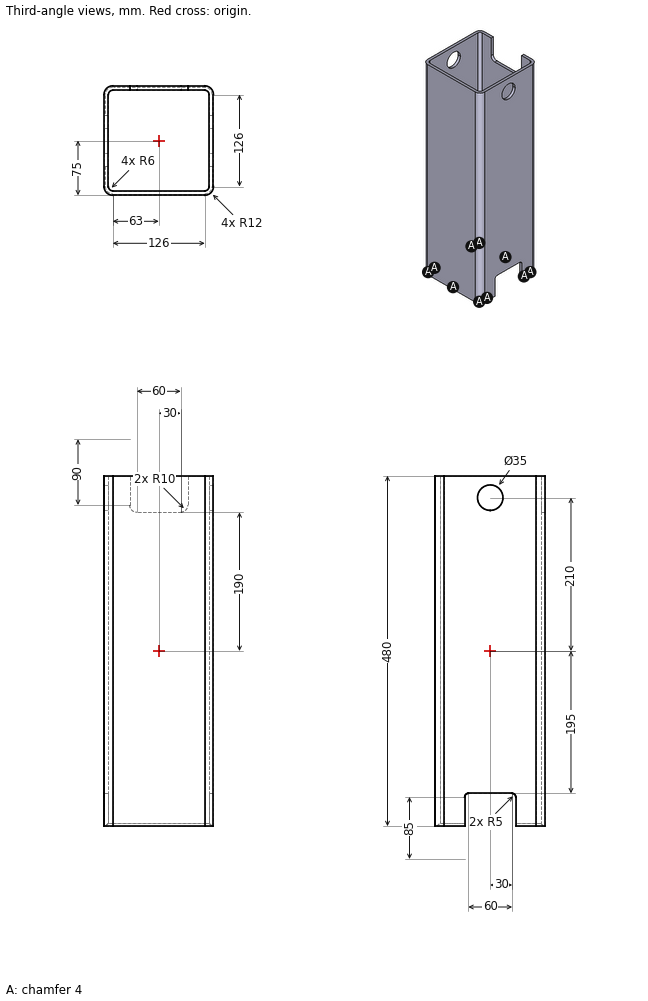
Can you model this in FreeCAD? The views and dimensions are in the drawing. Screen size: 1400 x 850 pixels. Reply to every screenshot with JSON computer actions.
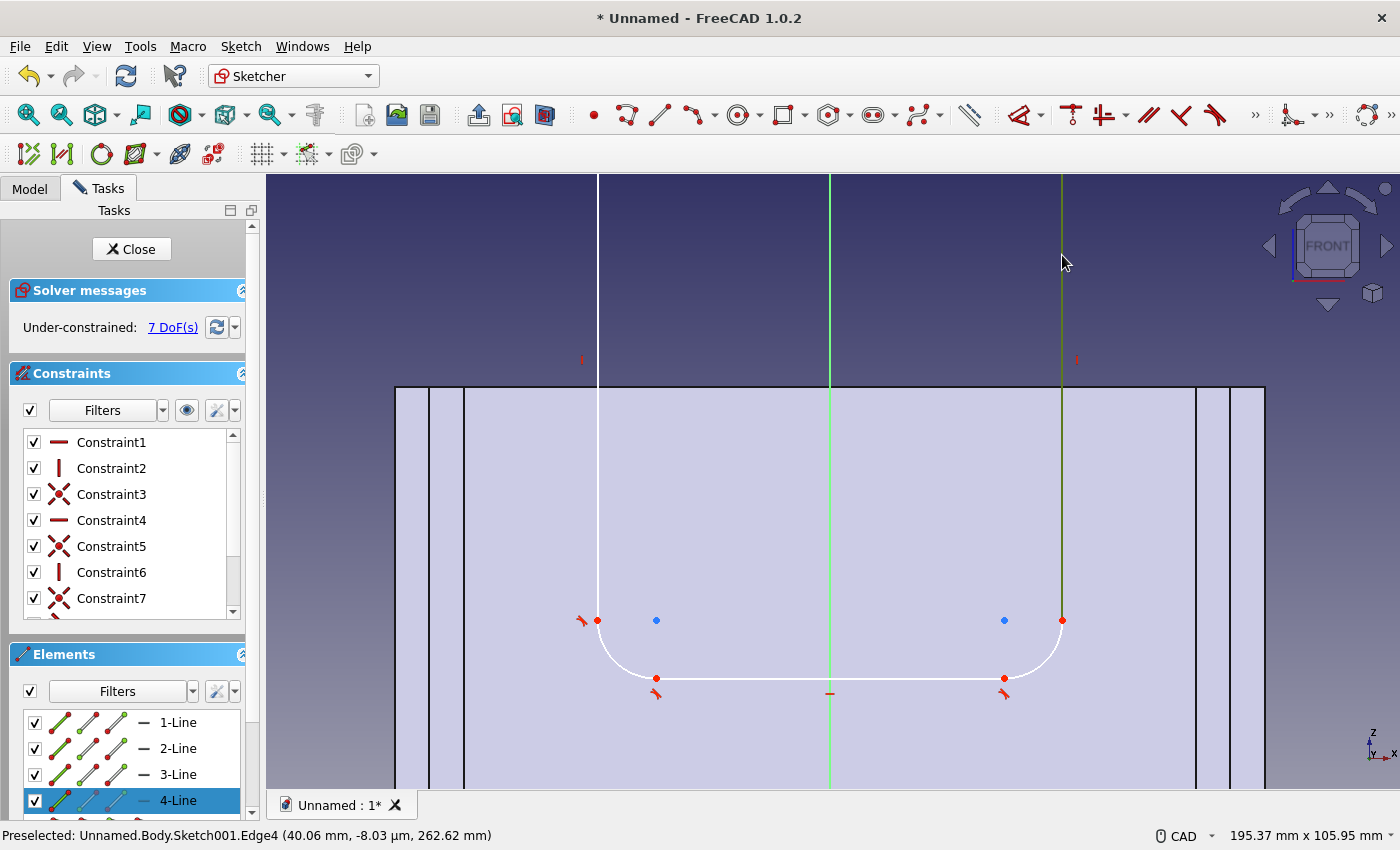
{"action": "left_click", "coordinate": [1031, 672]}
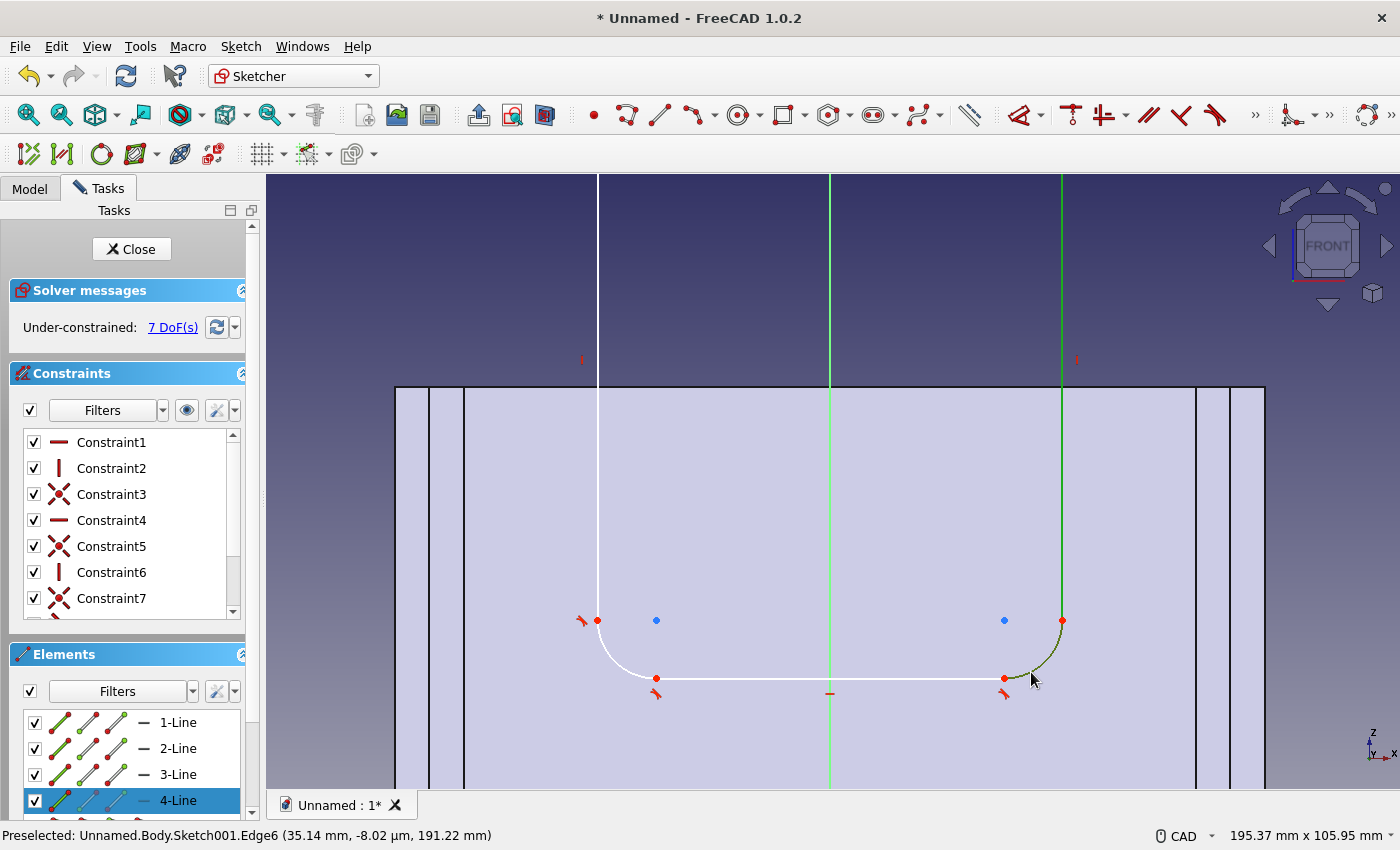
{"action": "key", "text": "t"}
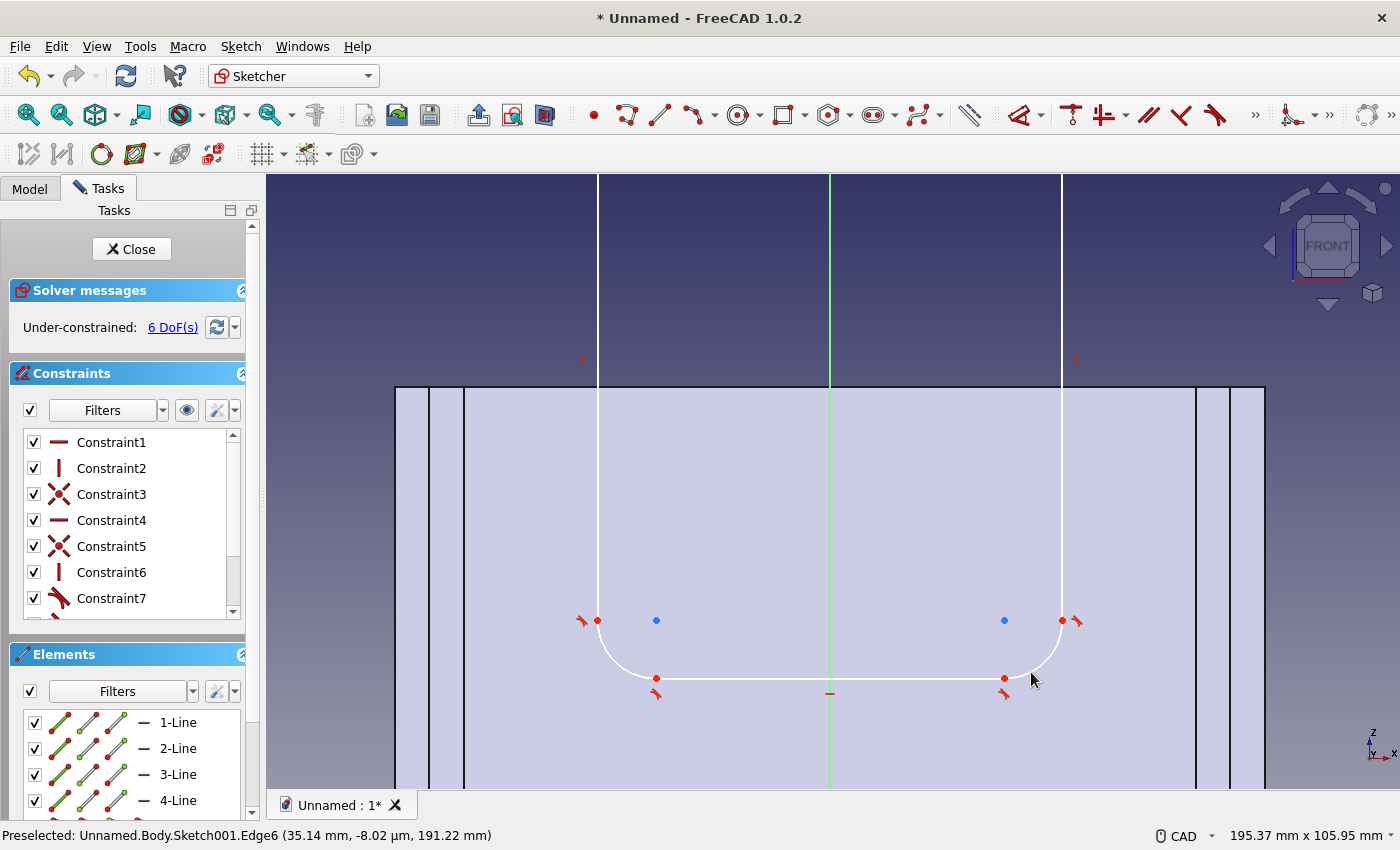
{"action": "left_click", "coordinate": [604, 647]}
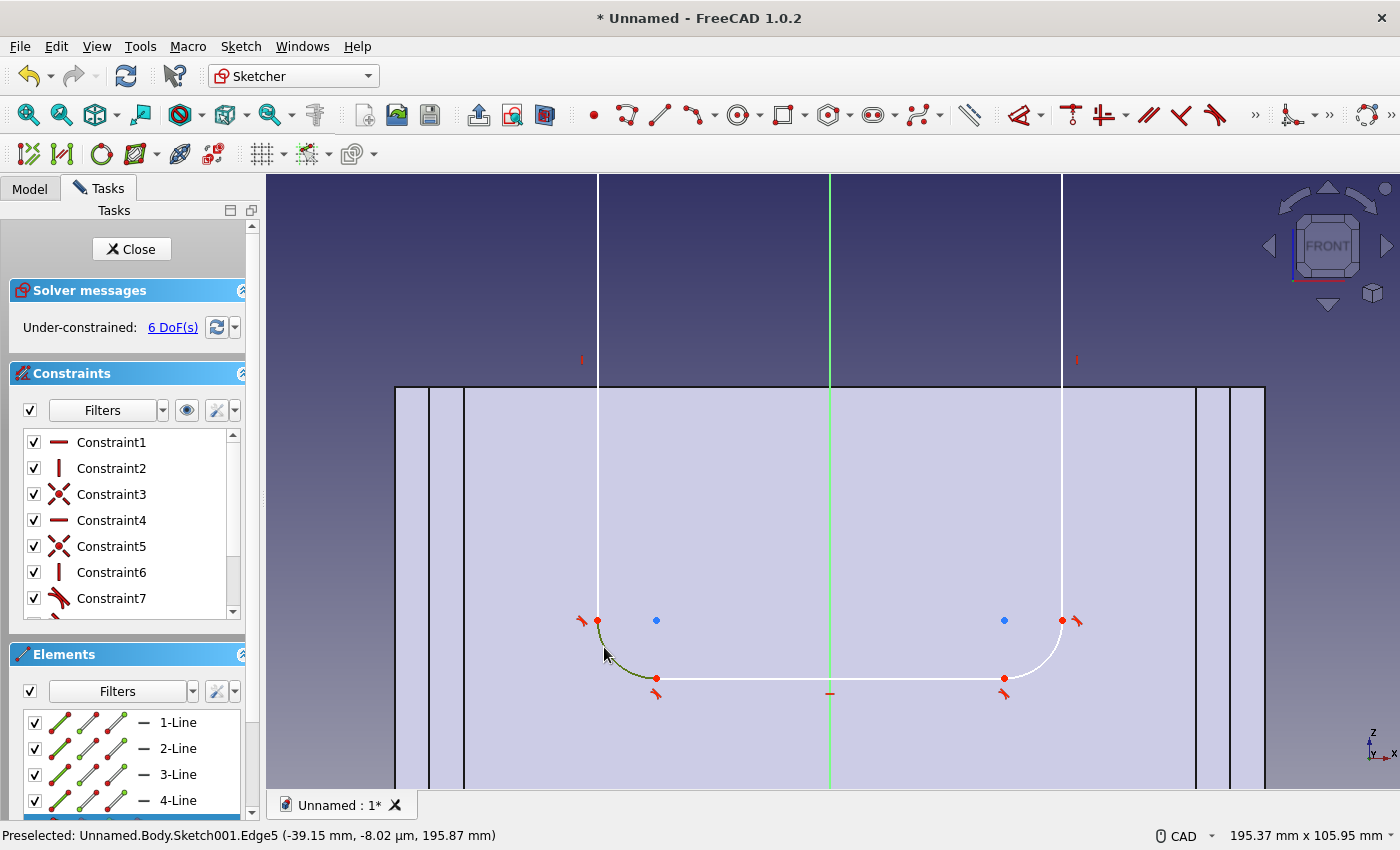
{"action": "left_click", "coordinate": [1031, 672]}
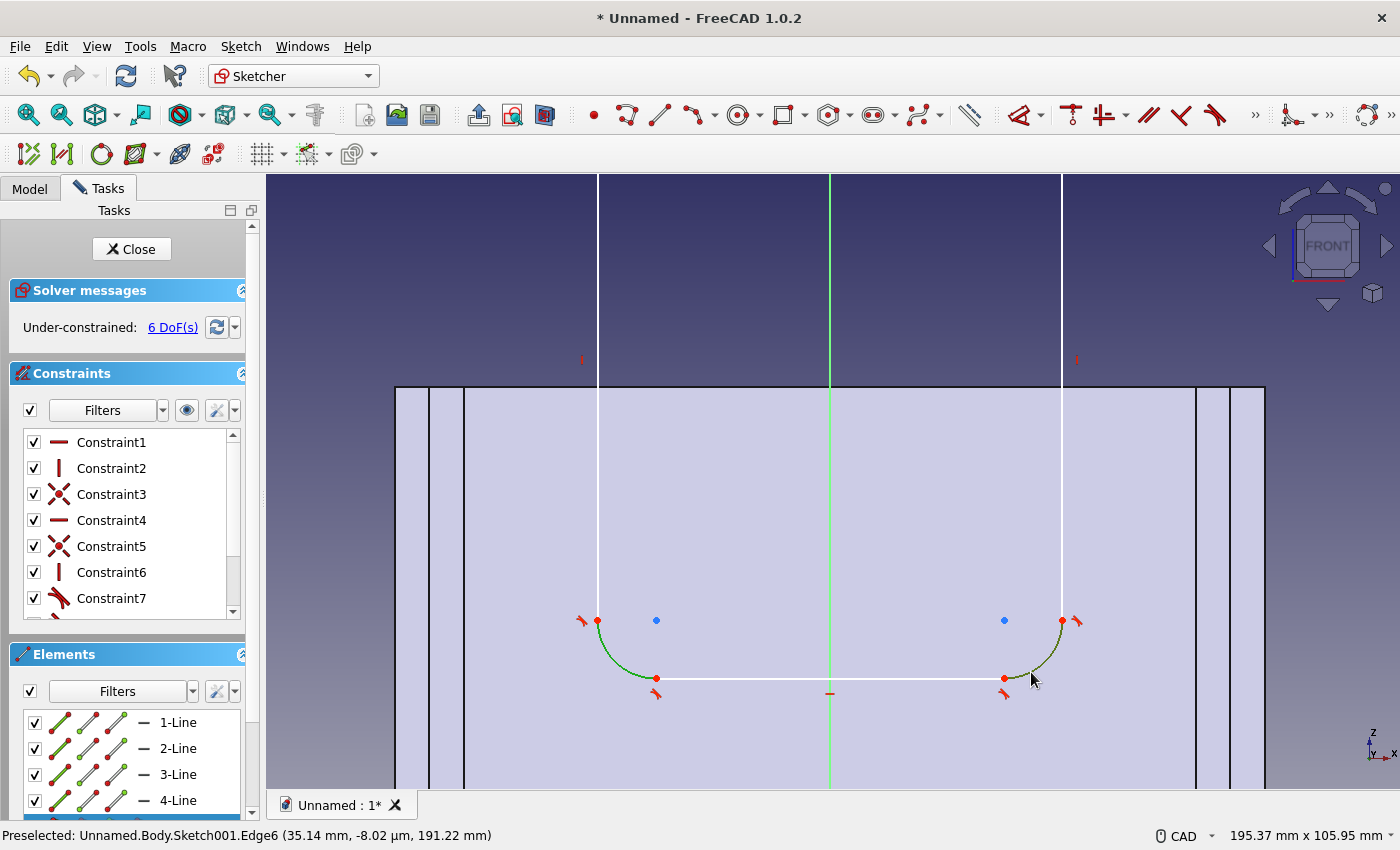
{"action": "key", "text": "e"}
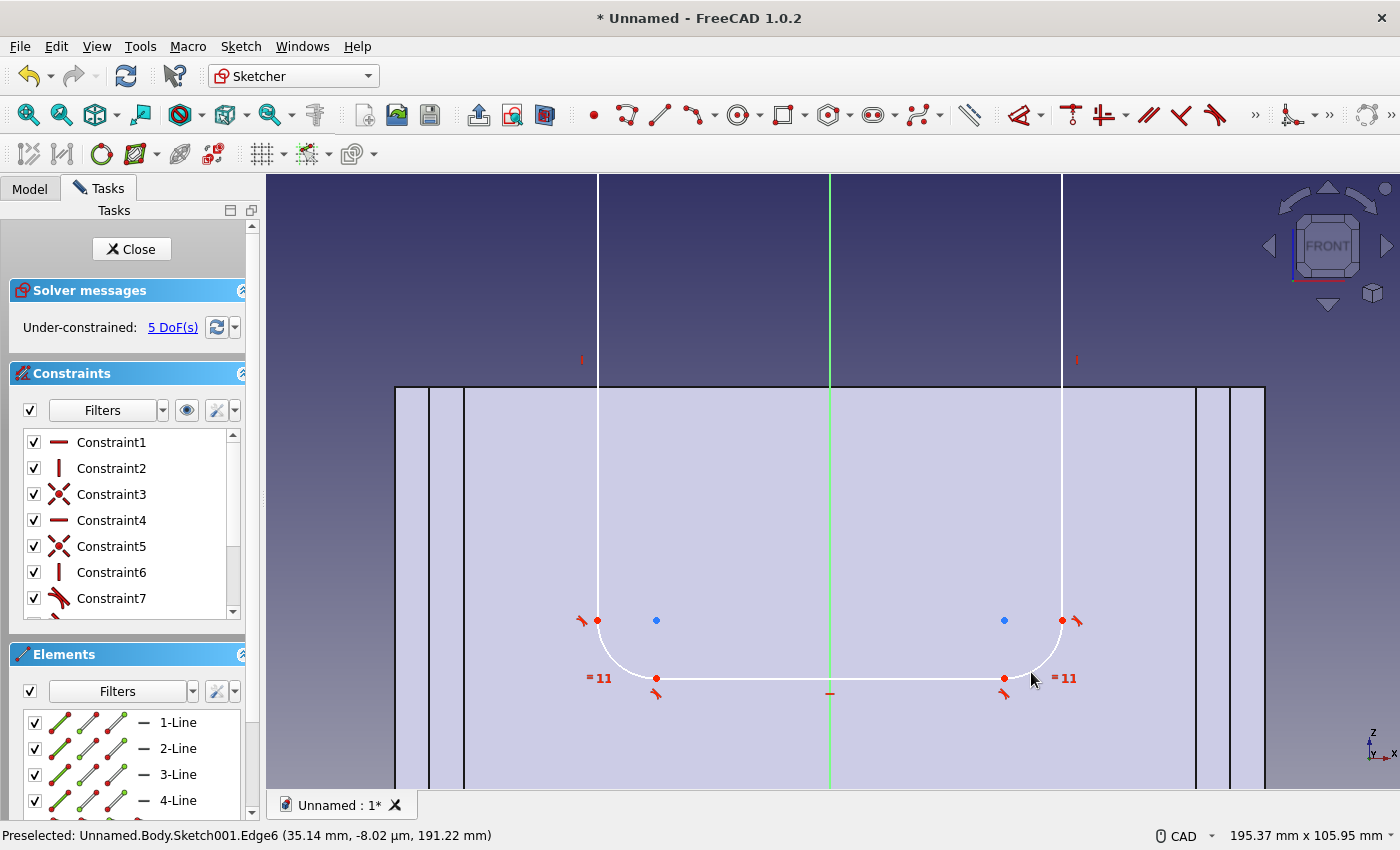
{"action": "left_click", "coordinate": [604, 647]}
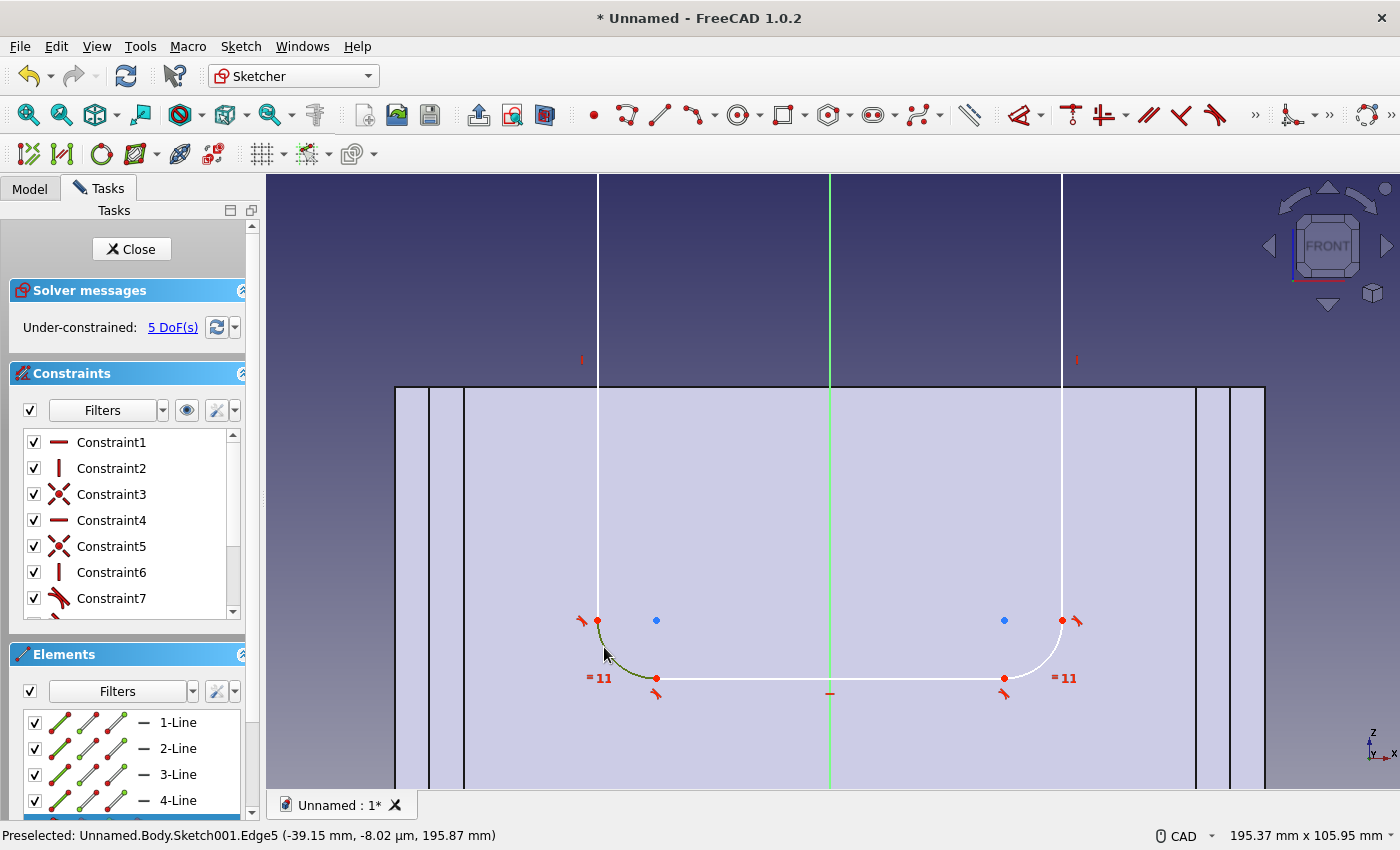
{"action": "key", "text": "k r"}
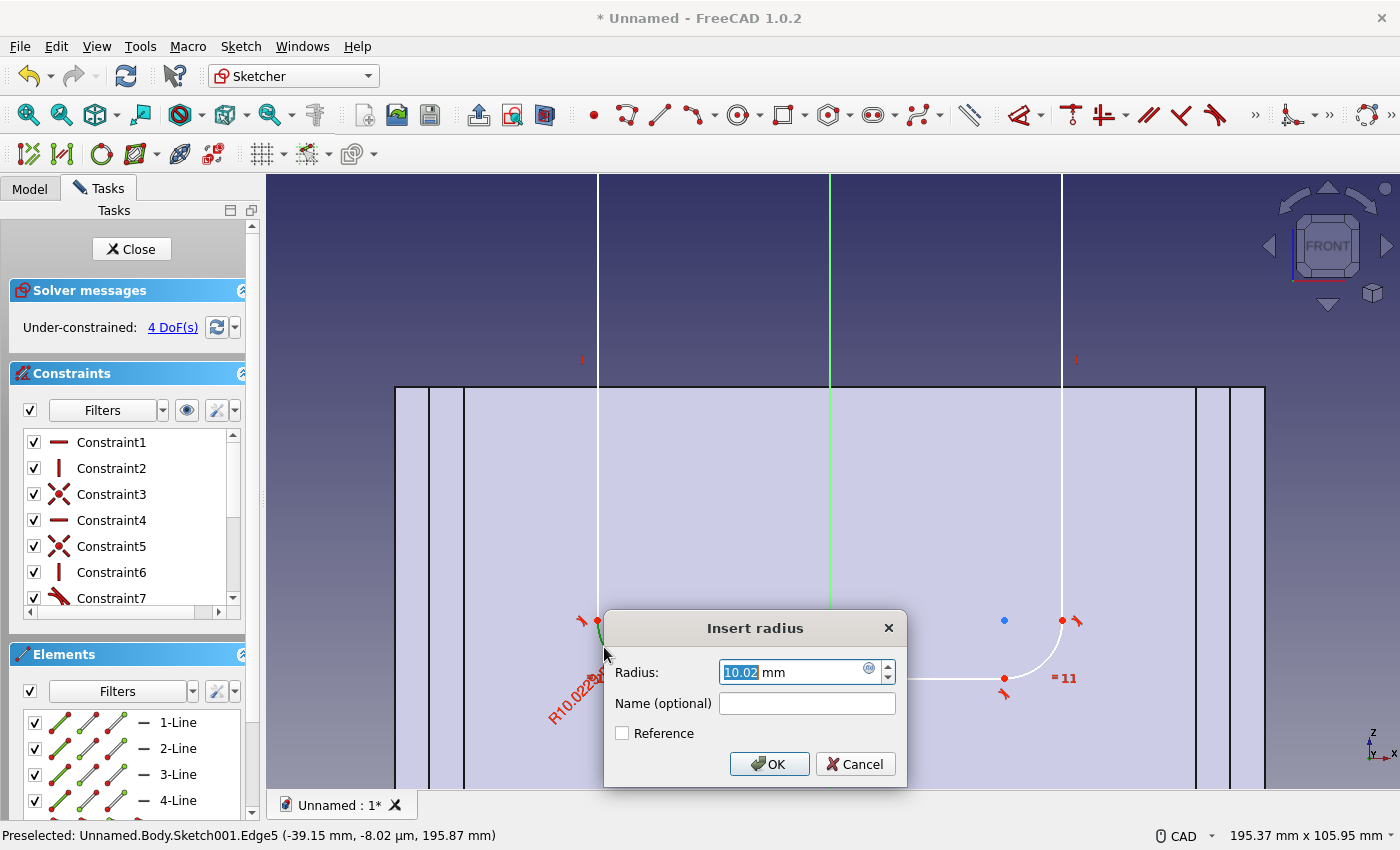
{"action": "type", "text": "10"}
{"action": "key", "text": "Return"}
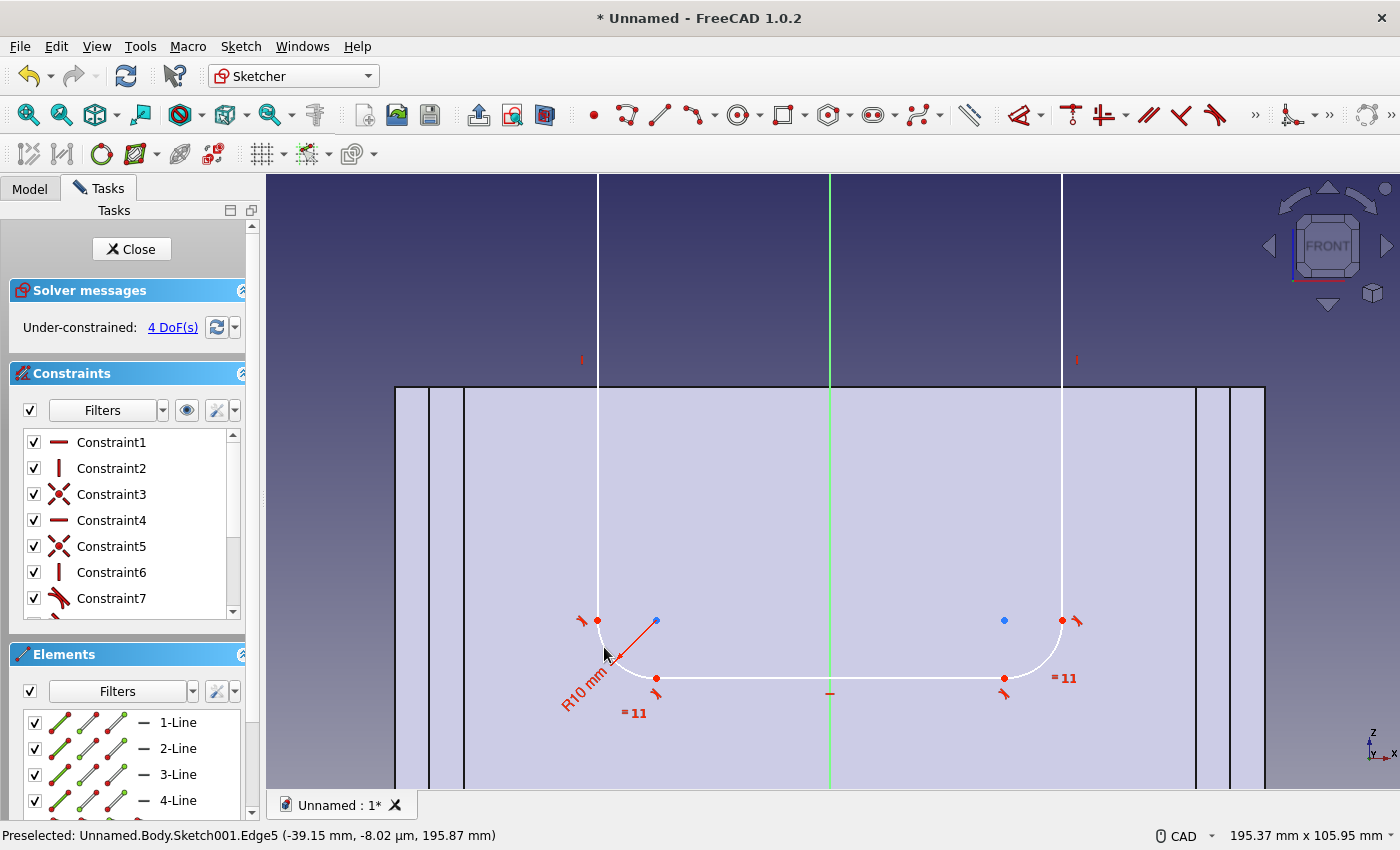
{"action": "left_click", "coordinate": [900, 678]}